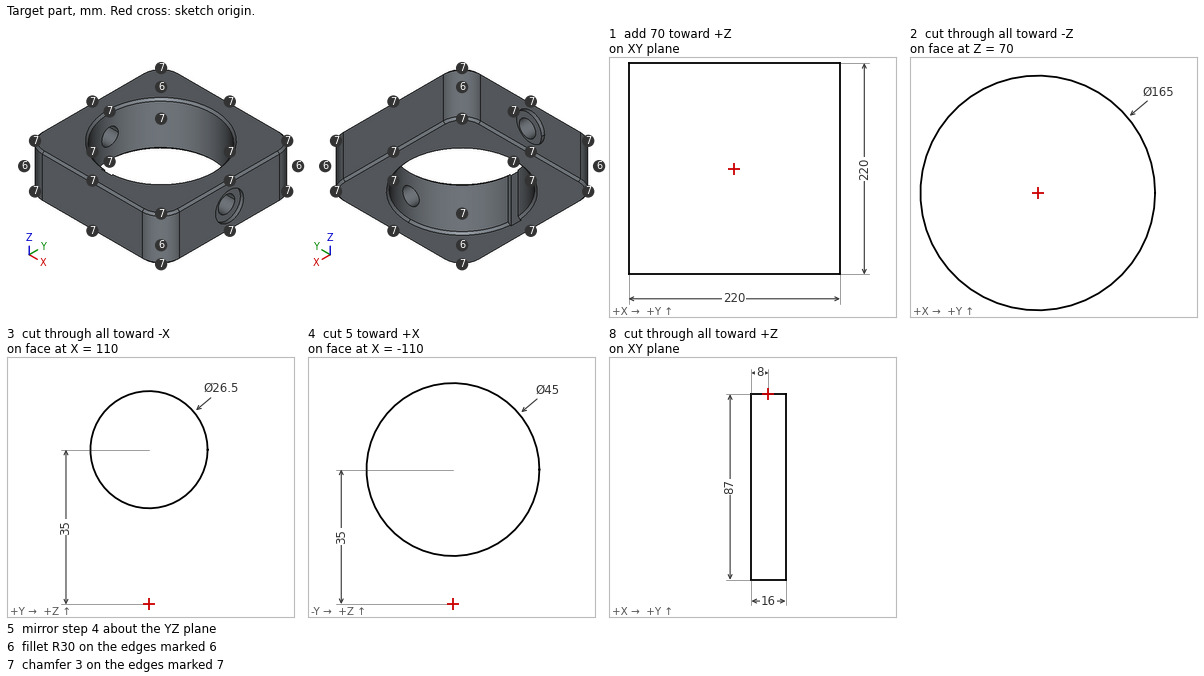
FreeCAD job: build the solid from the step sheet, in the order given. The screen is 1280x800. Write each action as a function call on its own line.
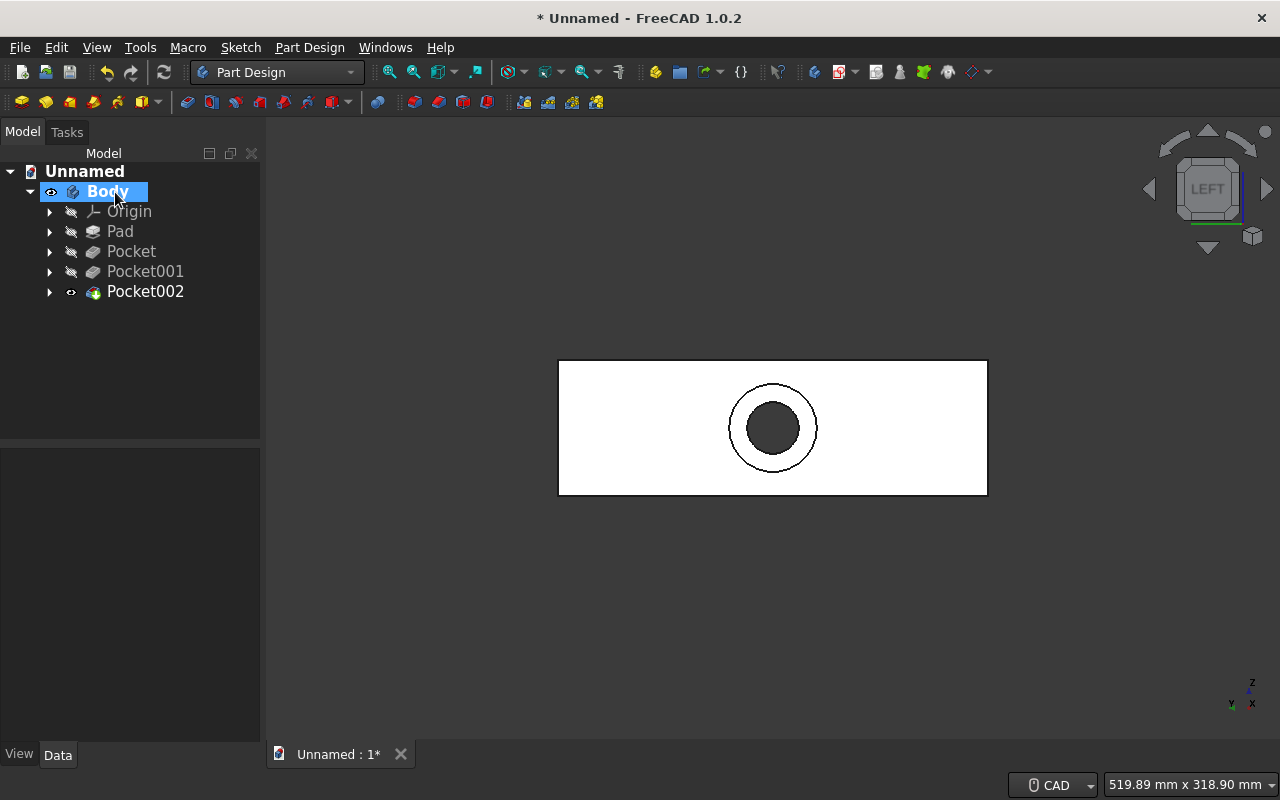
key(v)
key(f)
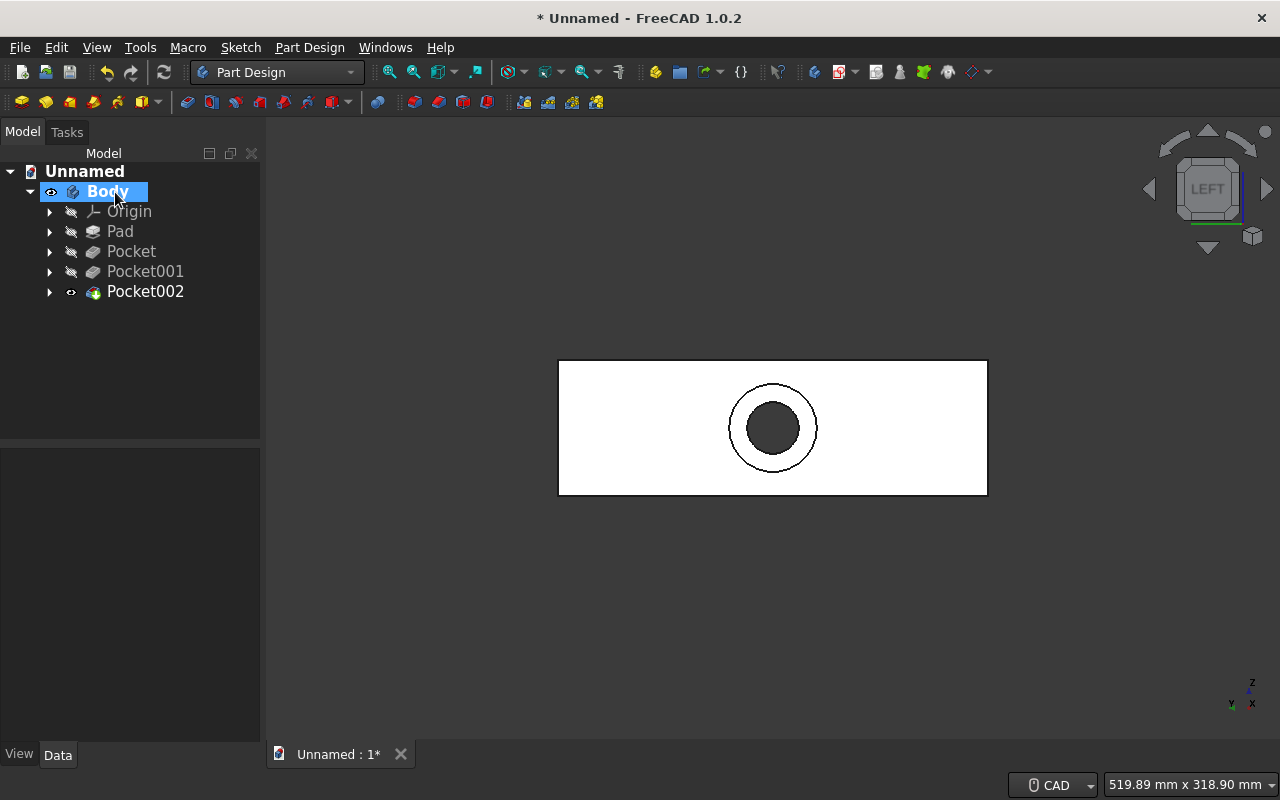
click(116, 292)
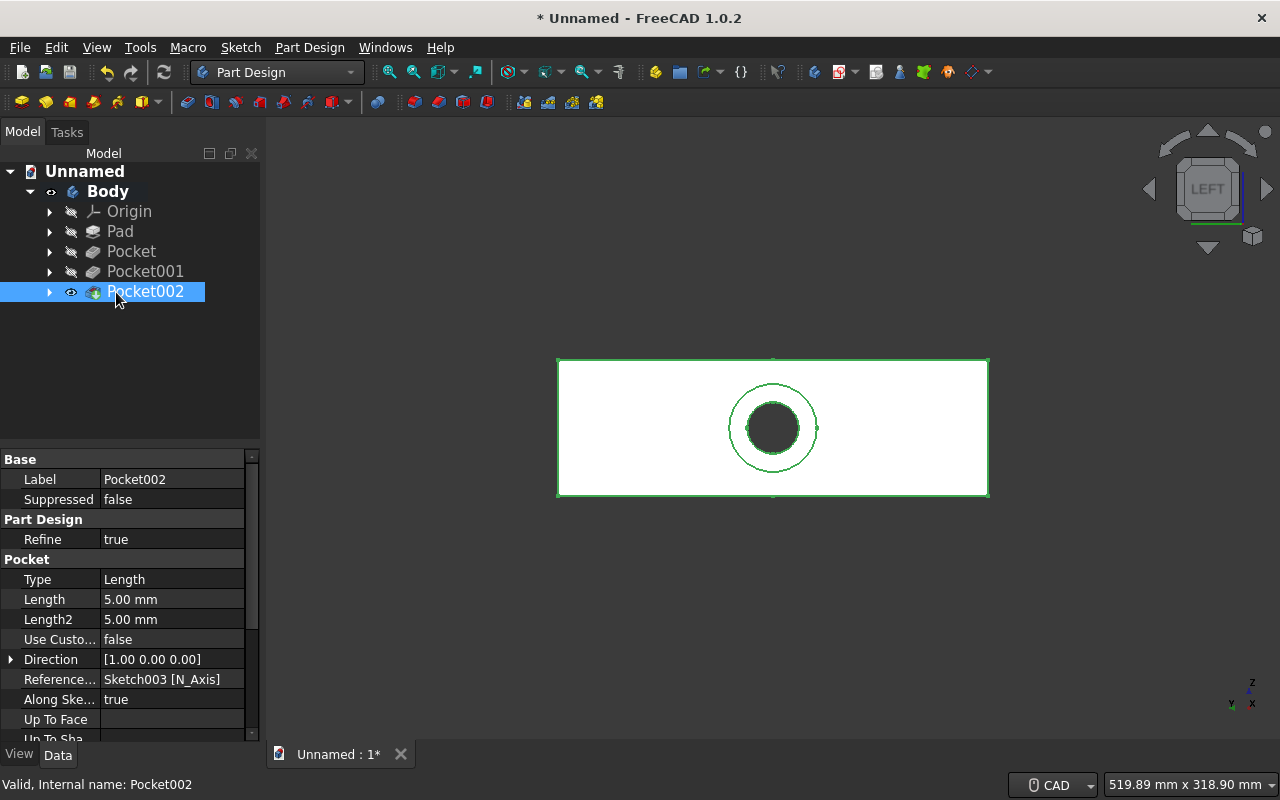
click(524, 102)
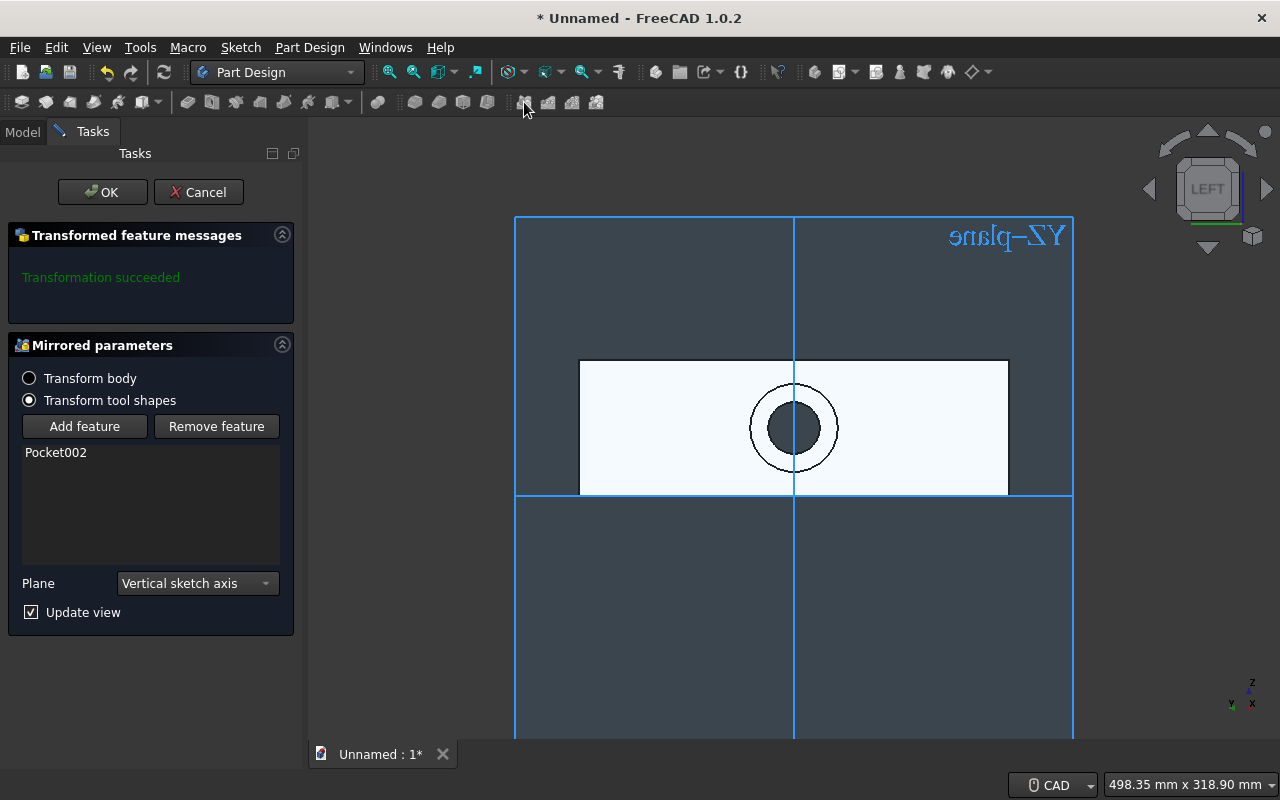
click(198, 584)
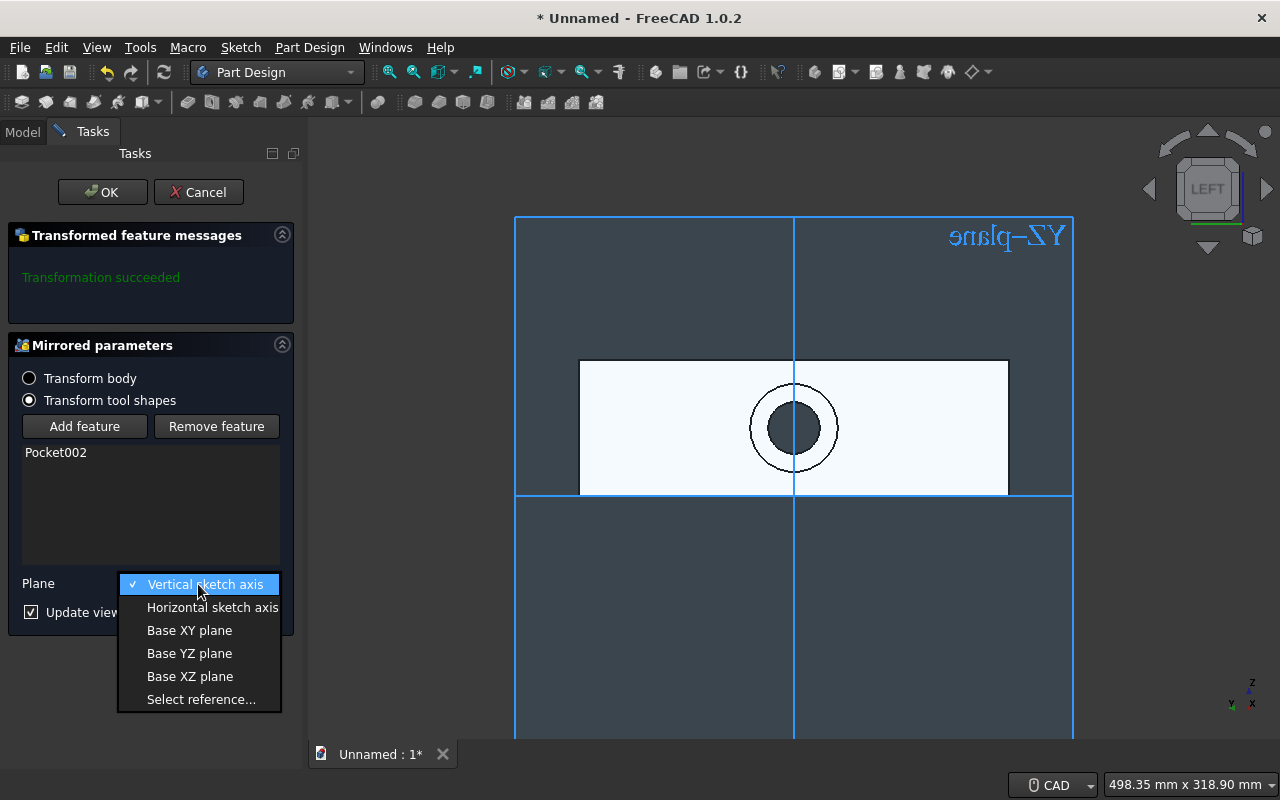
click(198, 654)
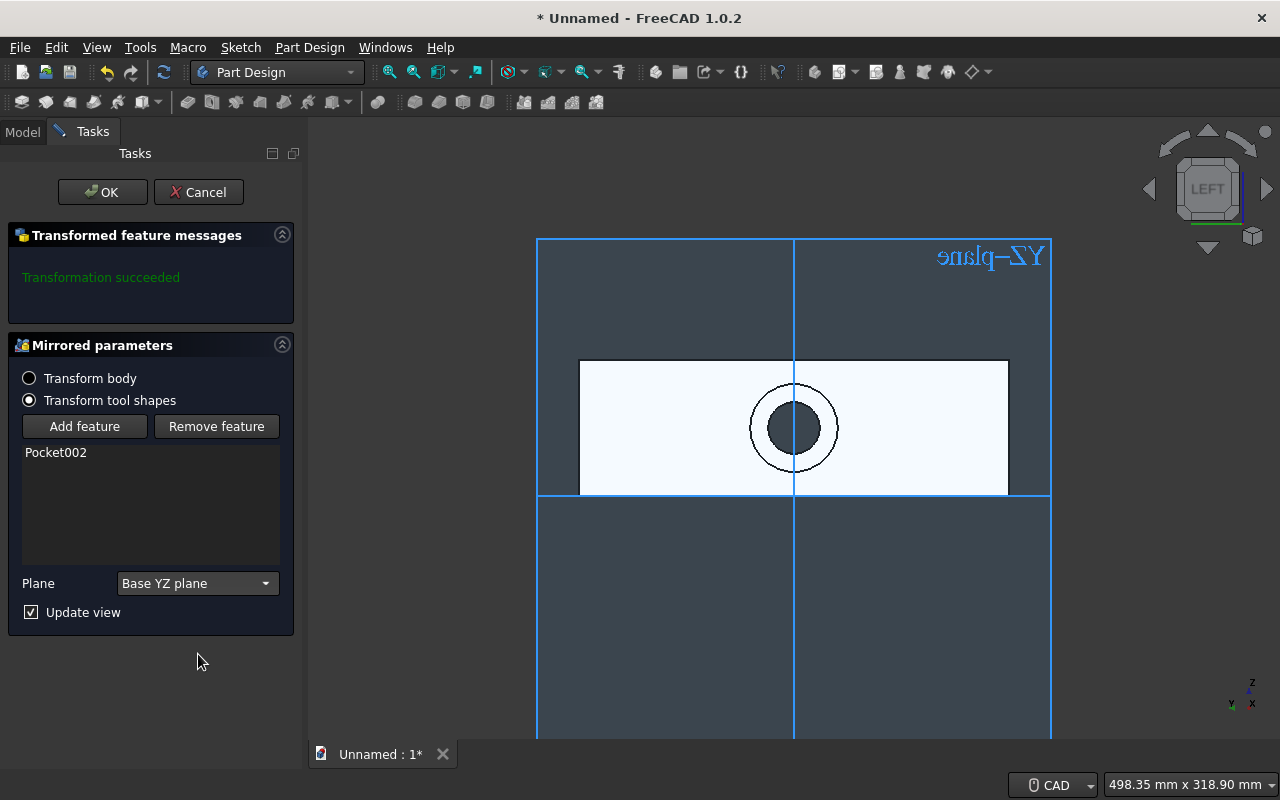
click(103, 192)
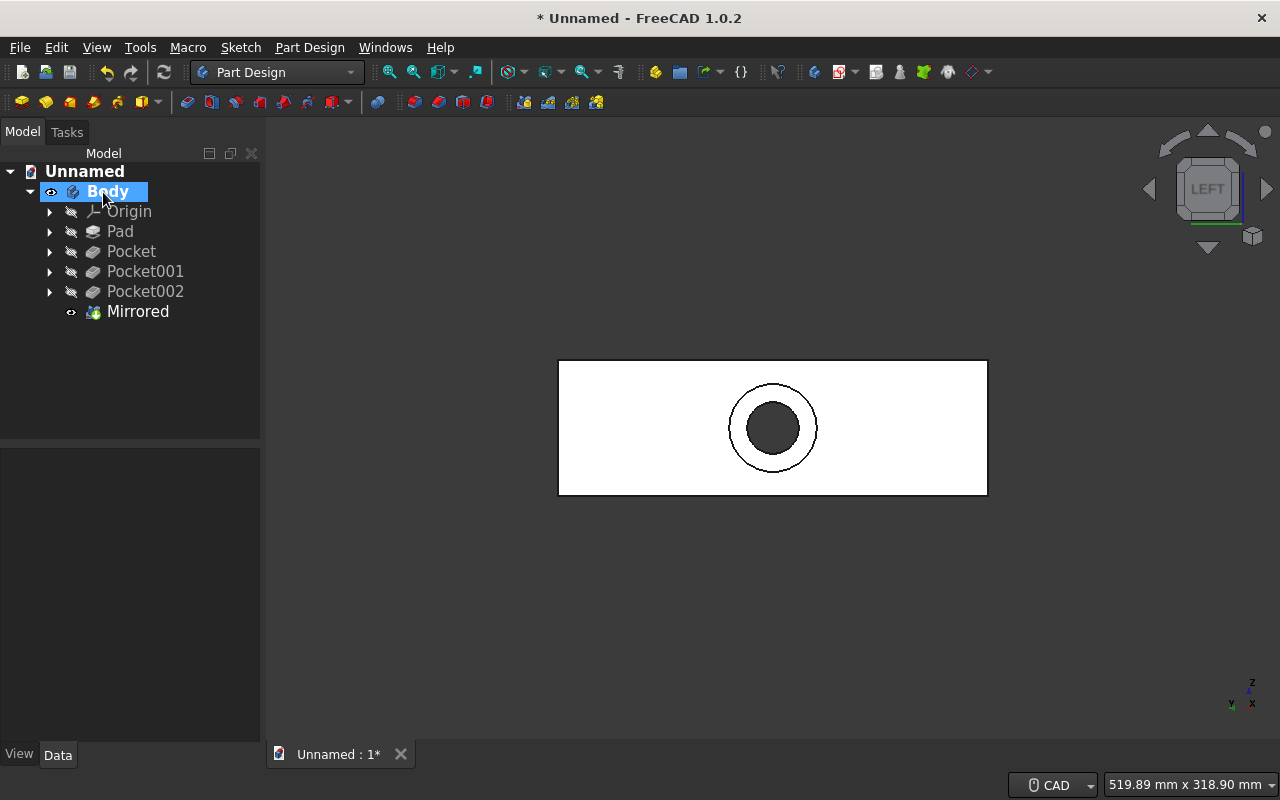
click(390, 72)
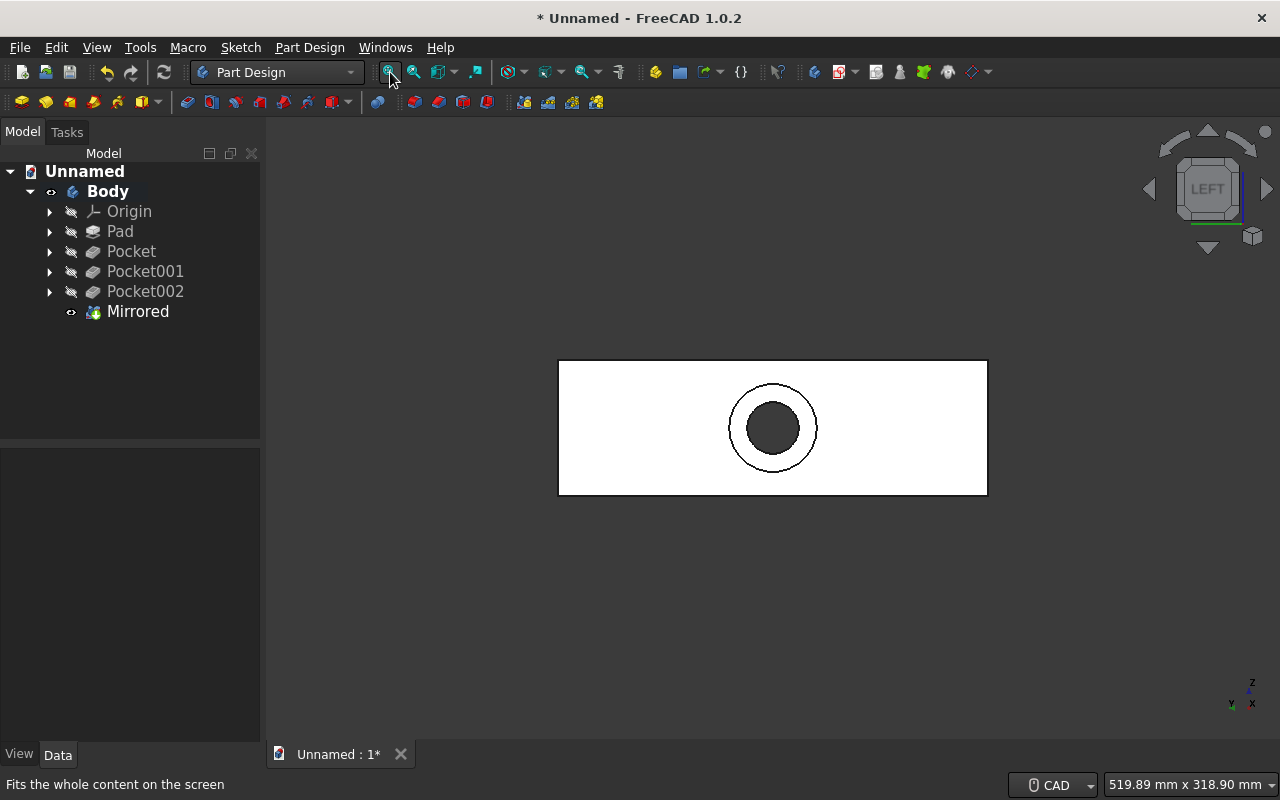
click(558, 427)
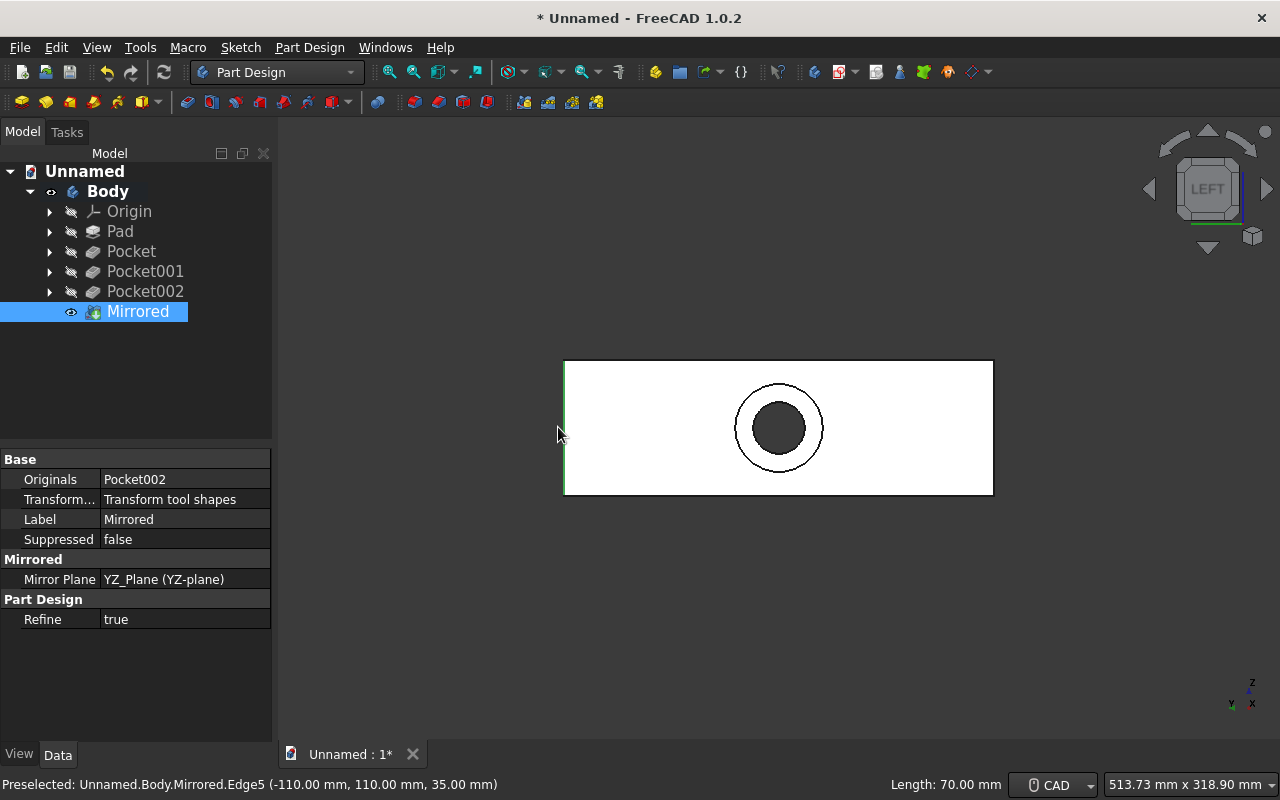
click(994, 427, ctrl)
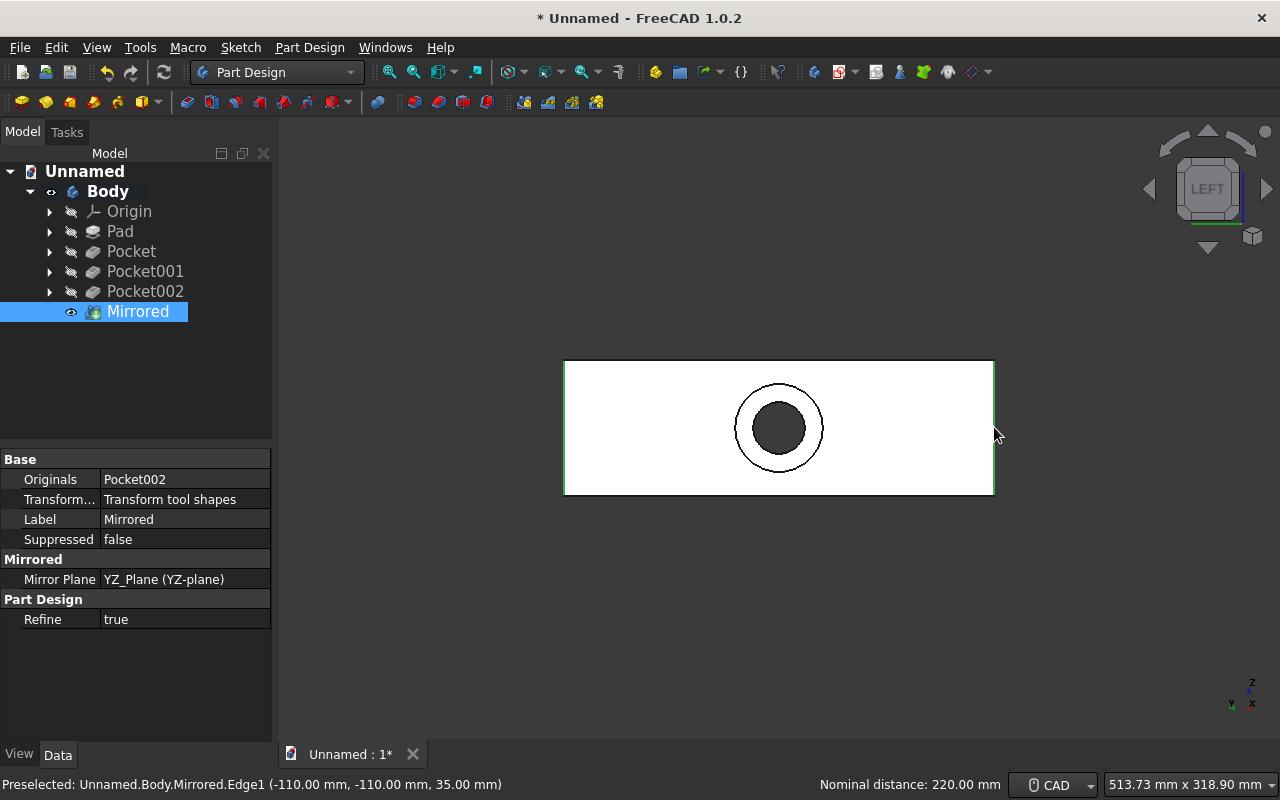
key(0)